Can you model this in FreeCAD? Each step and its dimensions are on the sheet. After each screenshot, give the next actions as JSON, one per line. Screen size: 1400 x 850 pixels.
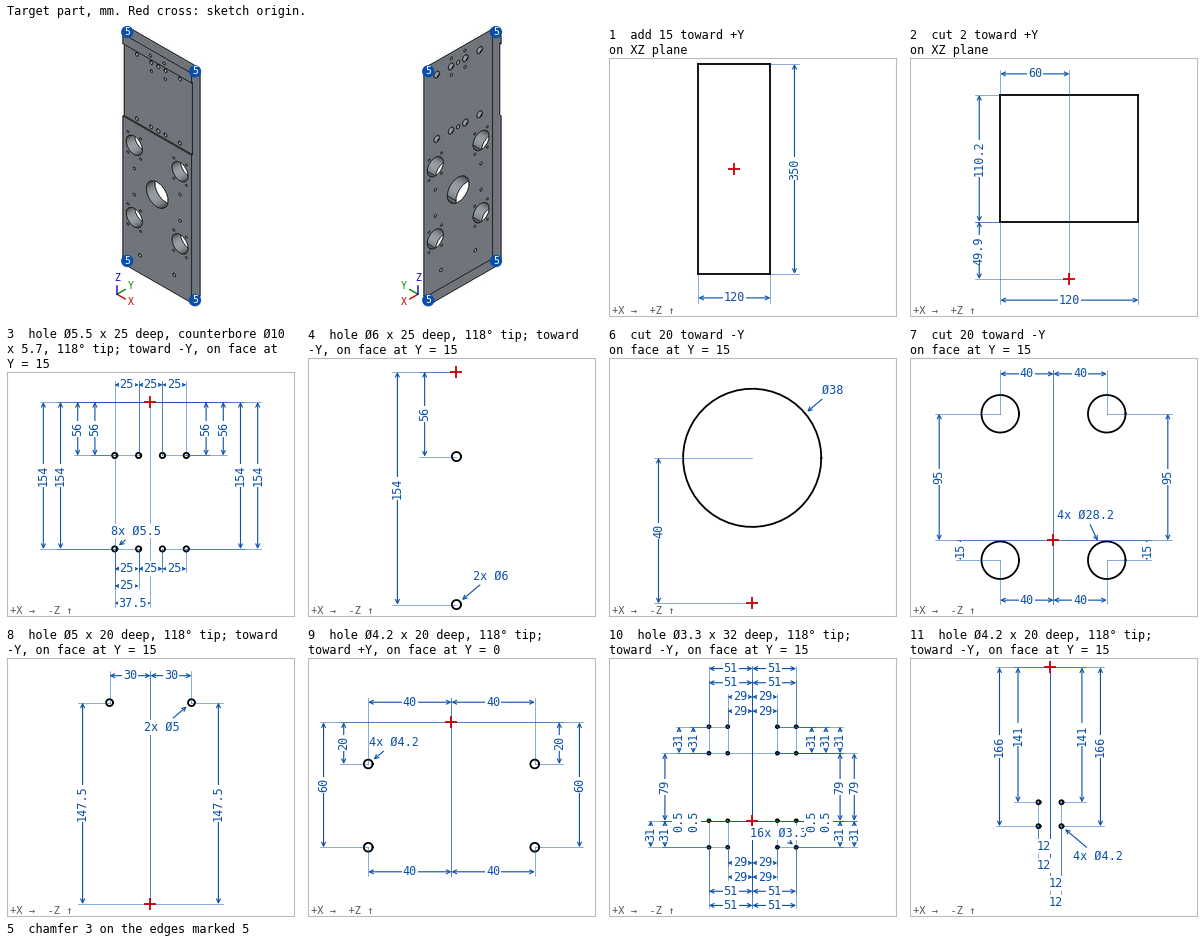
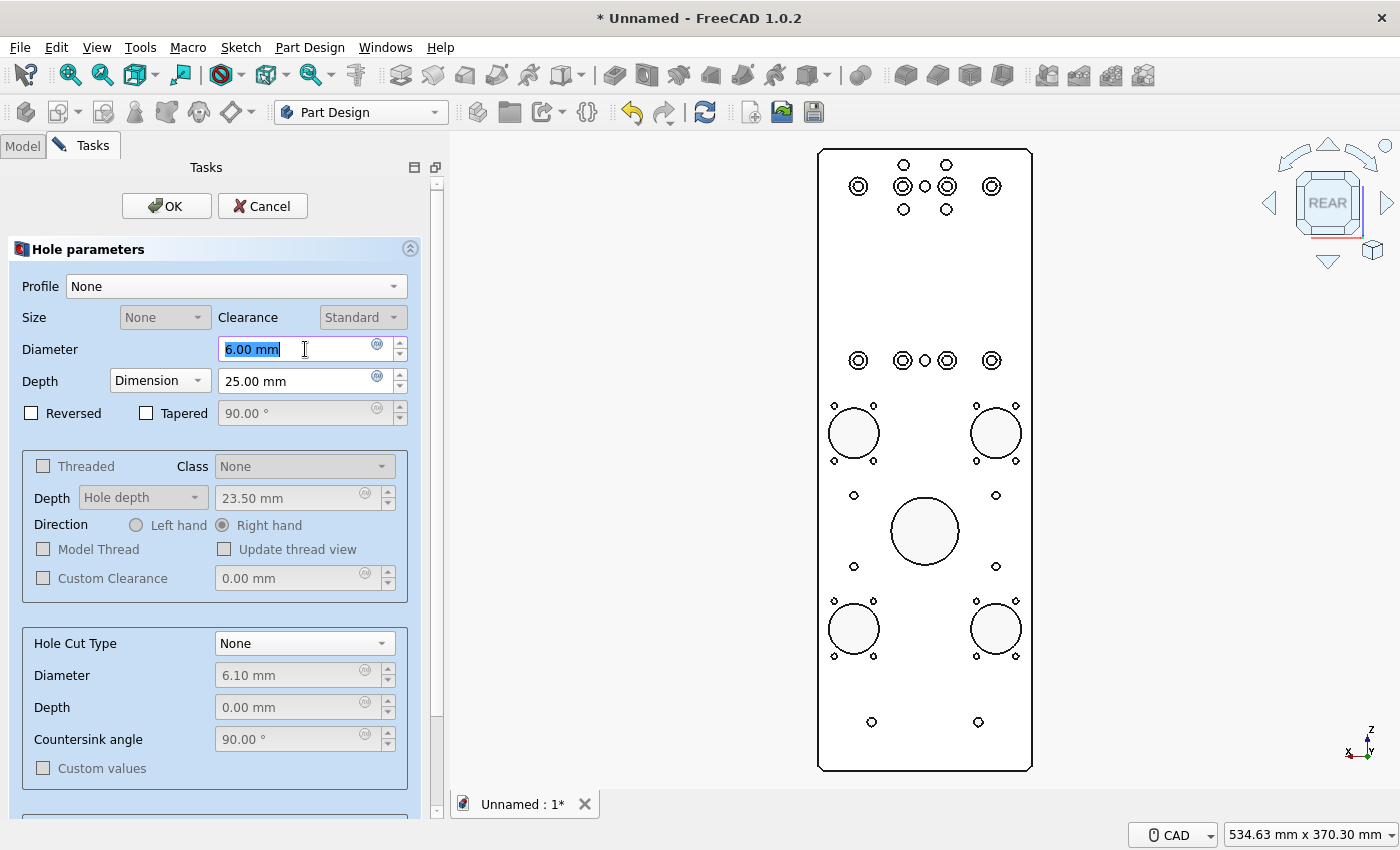
{"action": "type", "text": "4.2"}
{"action": "key", "text": "Tab"}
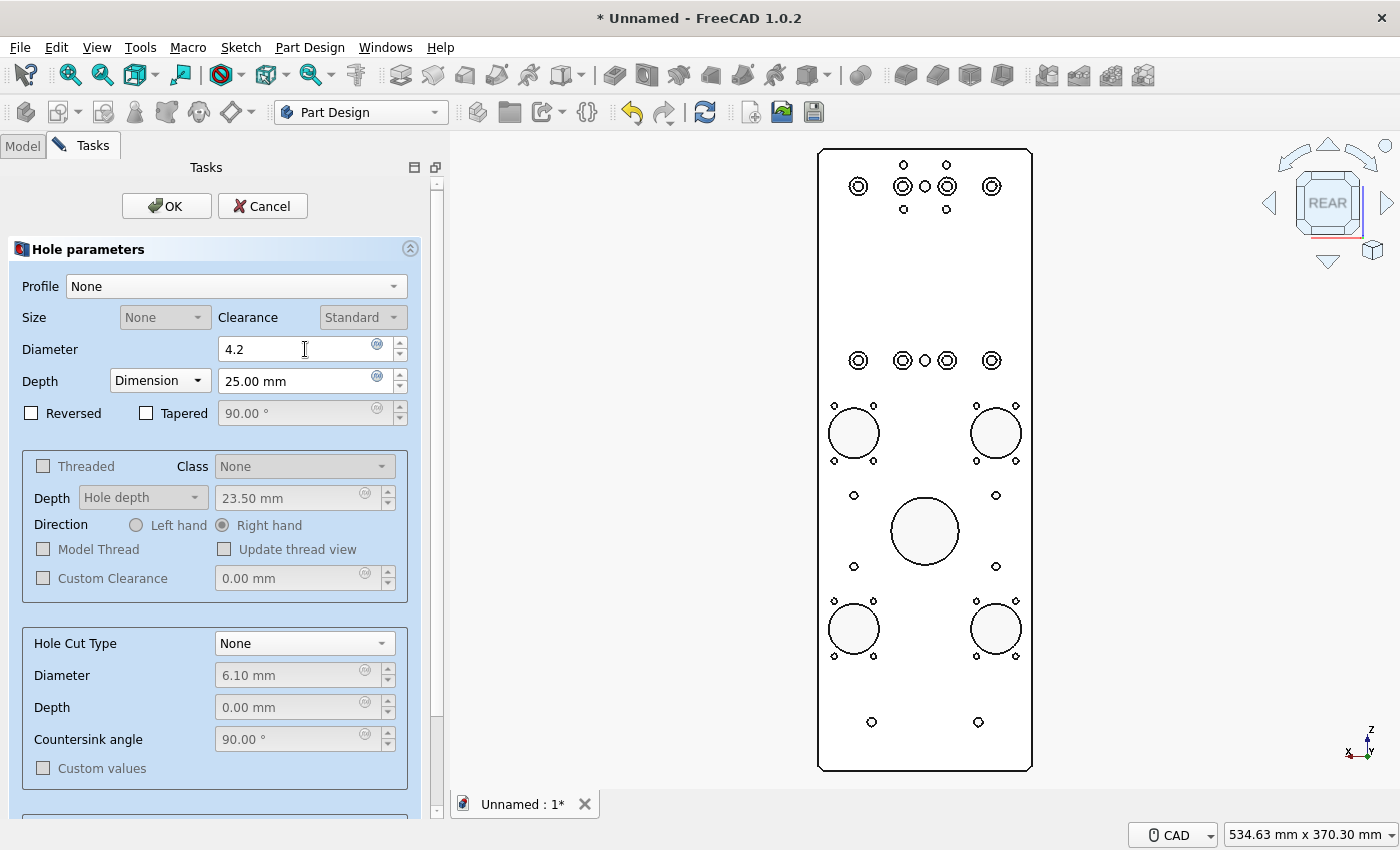
{"action": "triple_click", "coordinate": [305, 381]}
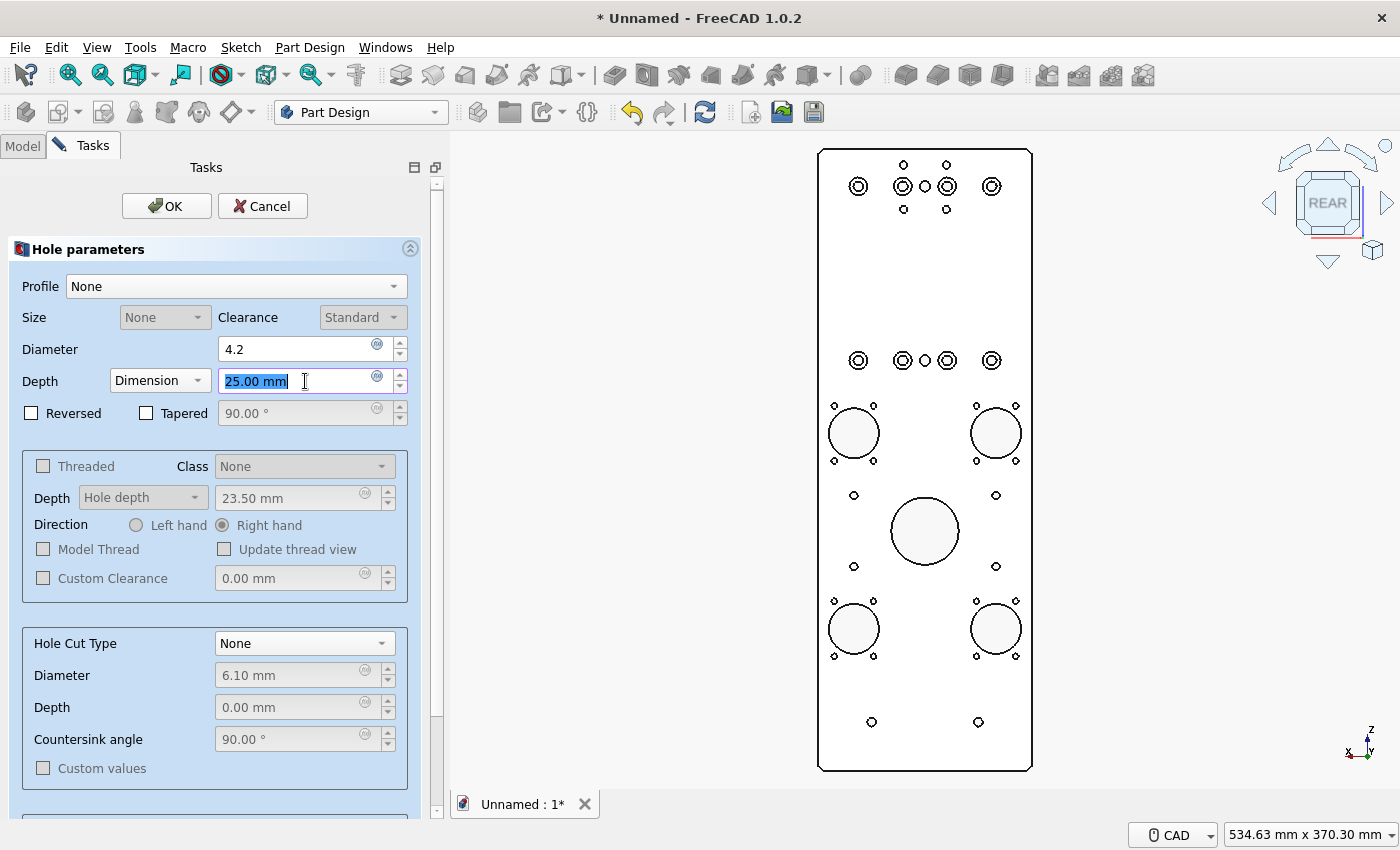
{"action": "type", "text": "20"}
{"action": "key", "text": "Tab"}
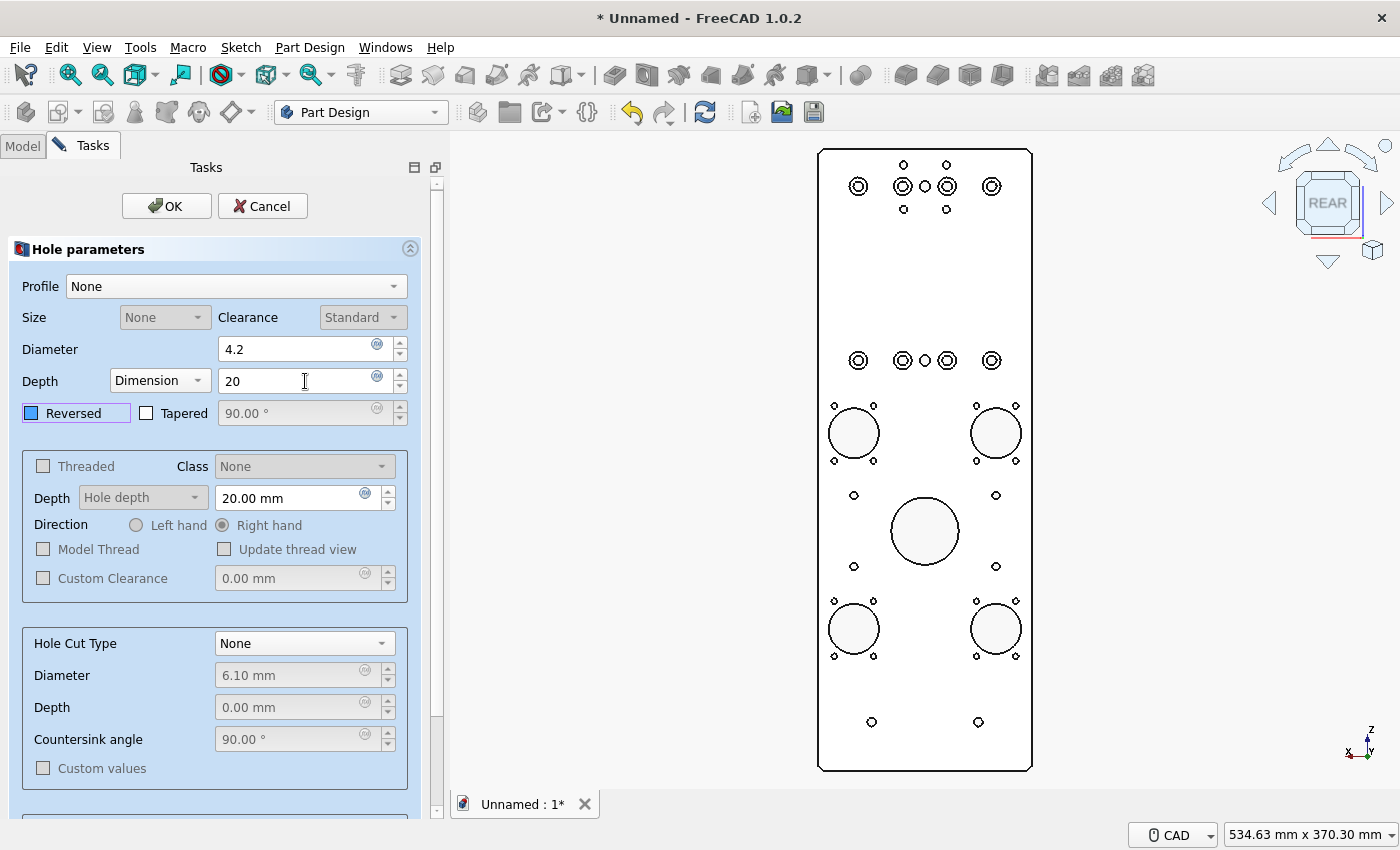
{"action": "left_click", "coordinate": [167, 206]}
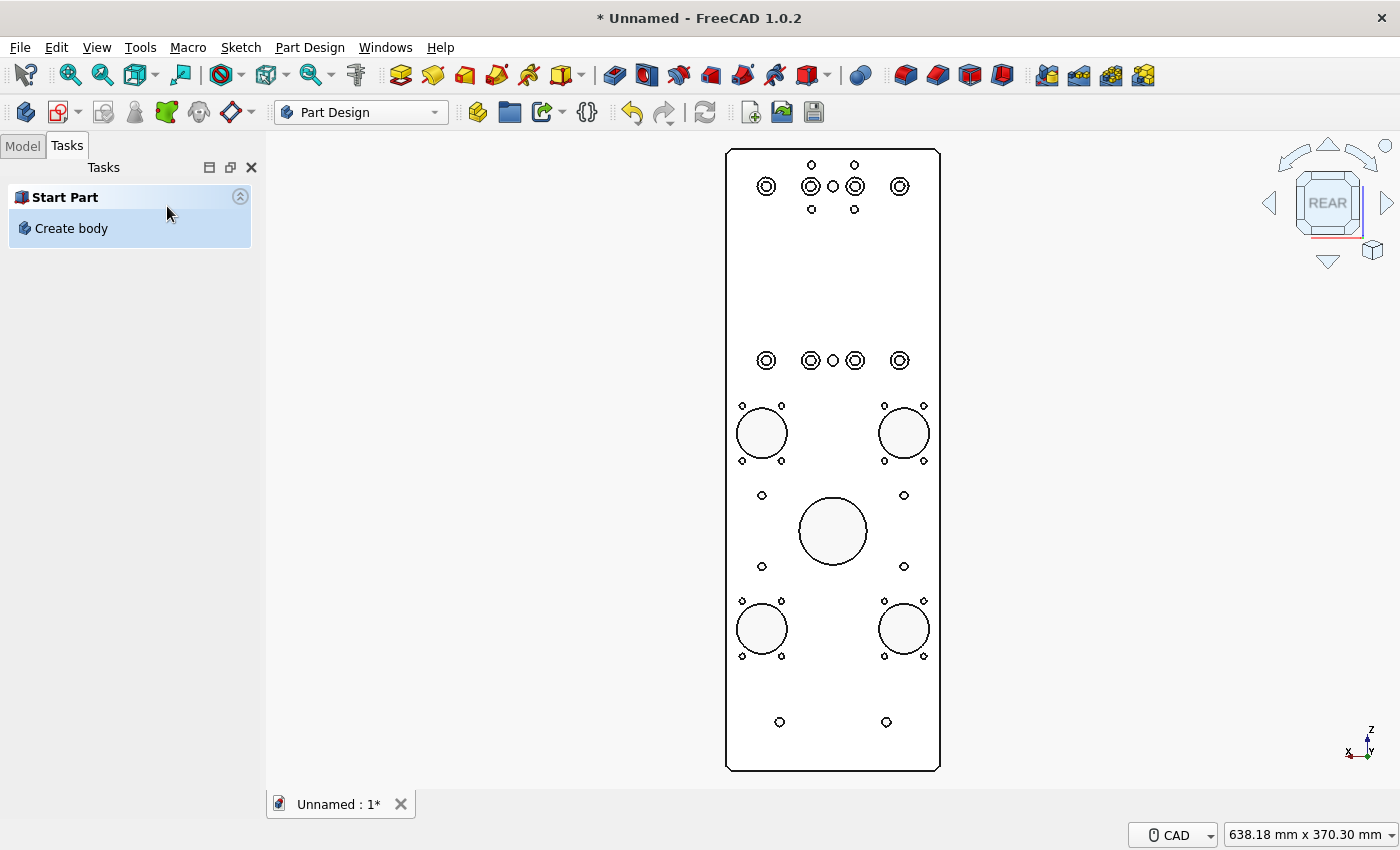
{"action": "key", "text": "0"}